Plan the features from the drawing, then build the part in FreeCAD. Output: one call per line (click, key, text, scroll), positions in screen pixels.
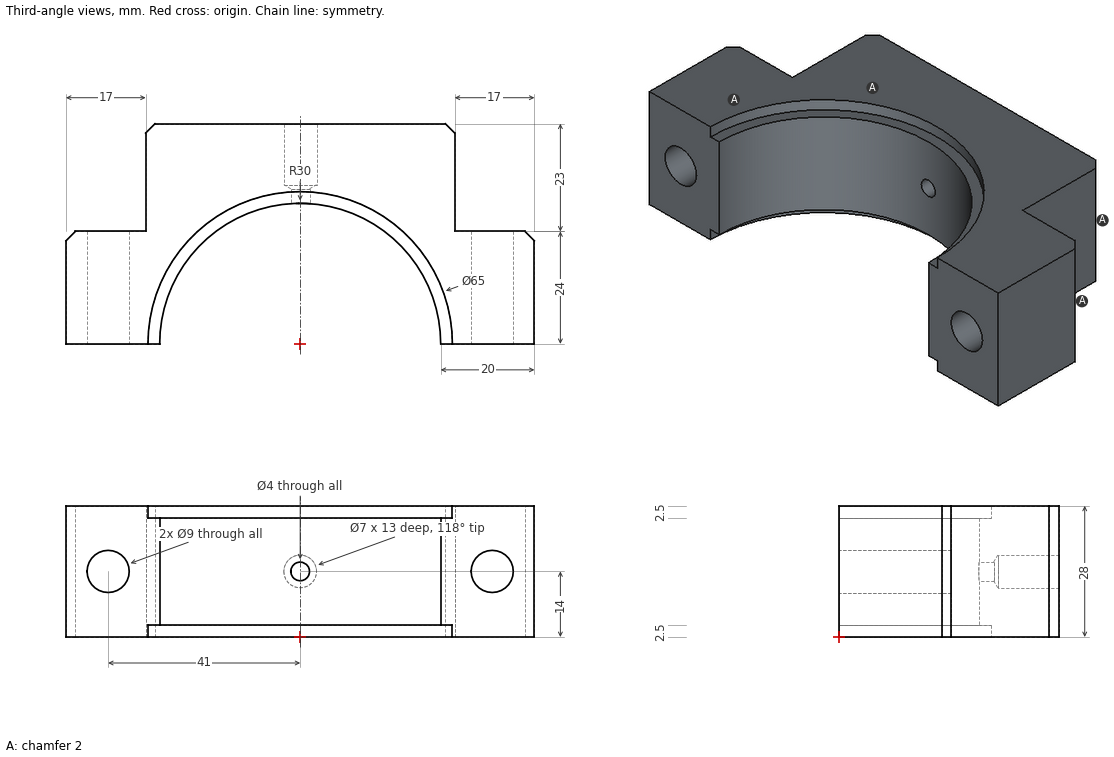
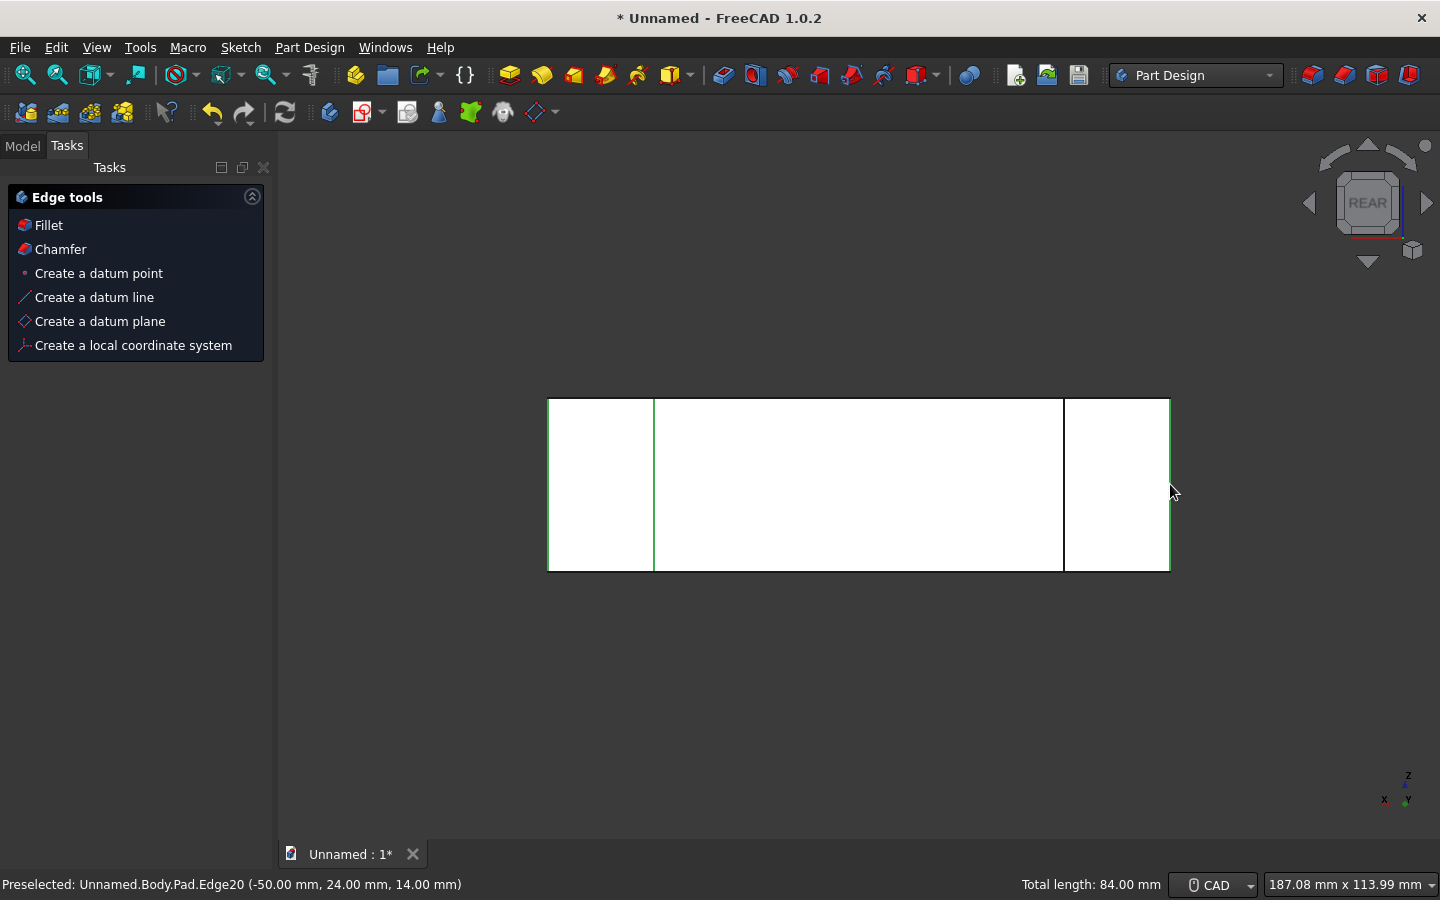
click(1064, 484, ctrl)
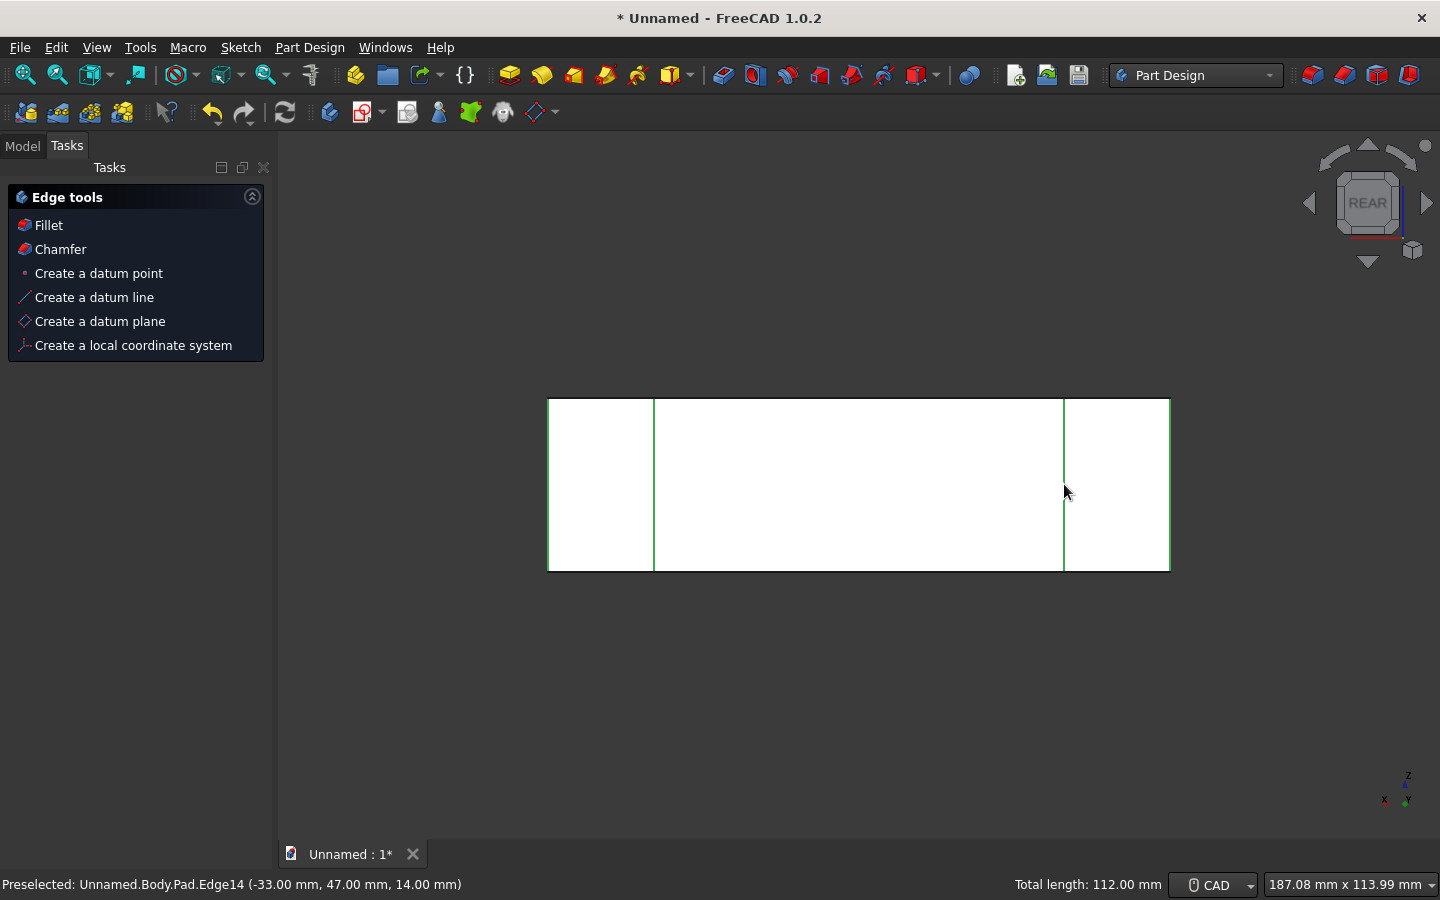
click(1346, 76)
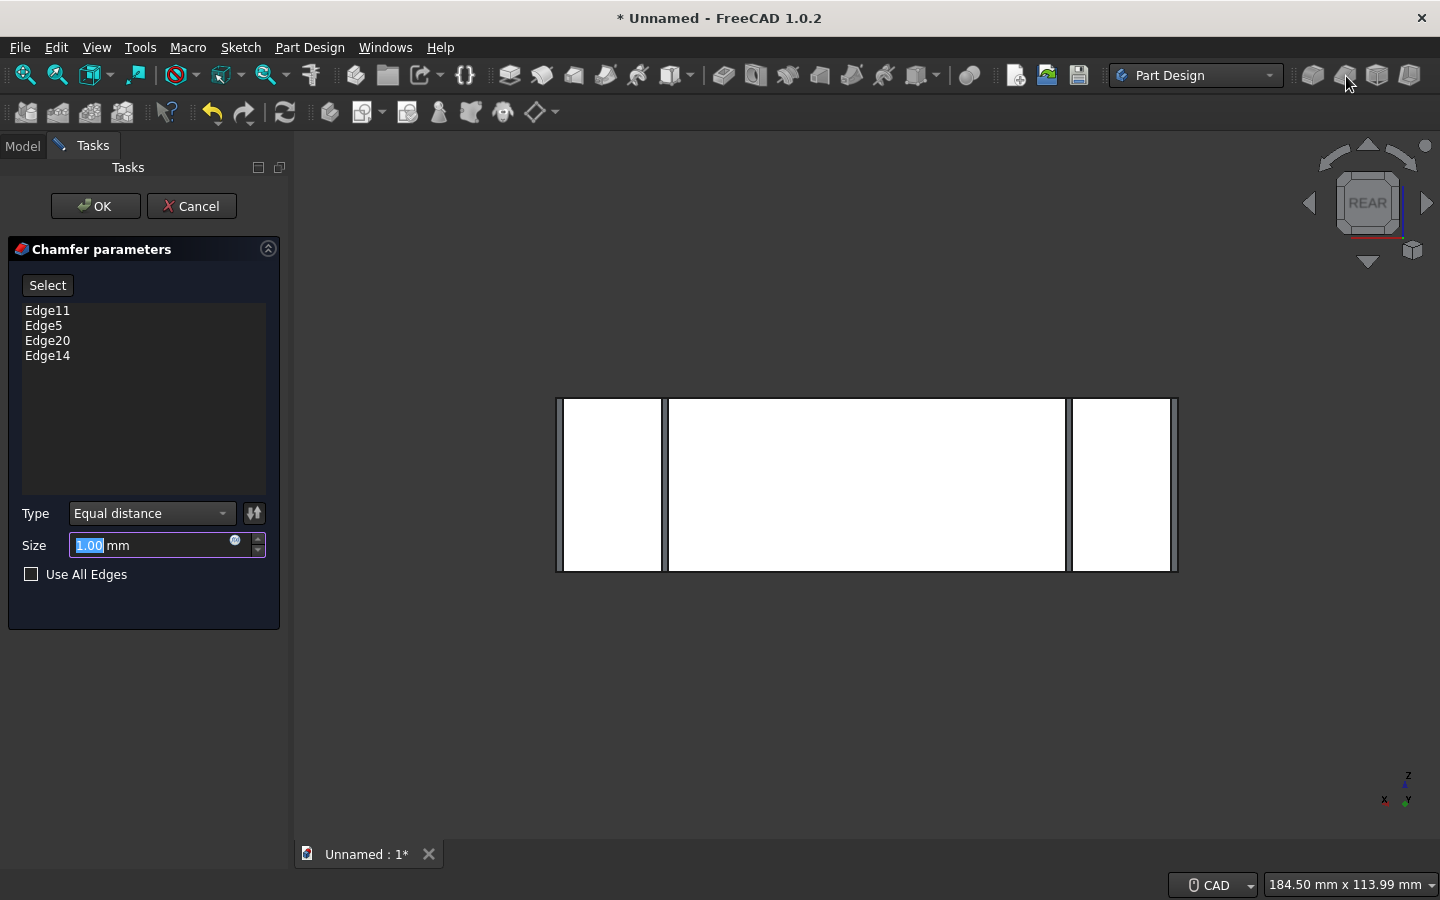
text(2)
key(Tab)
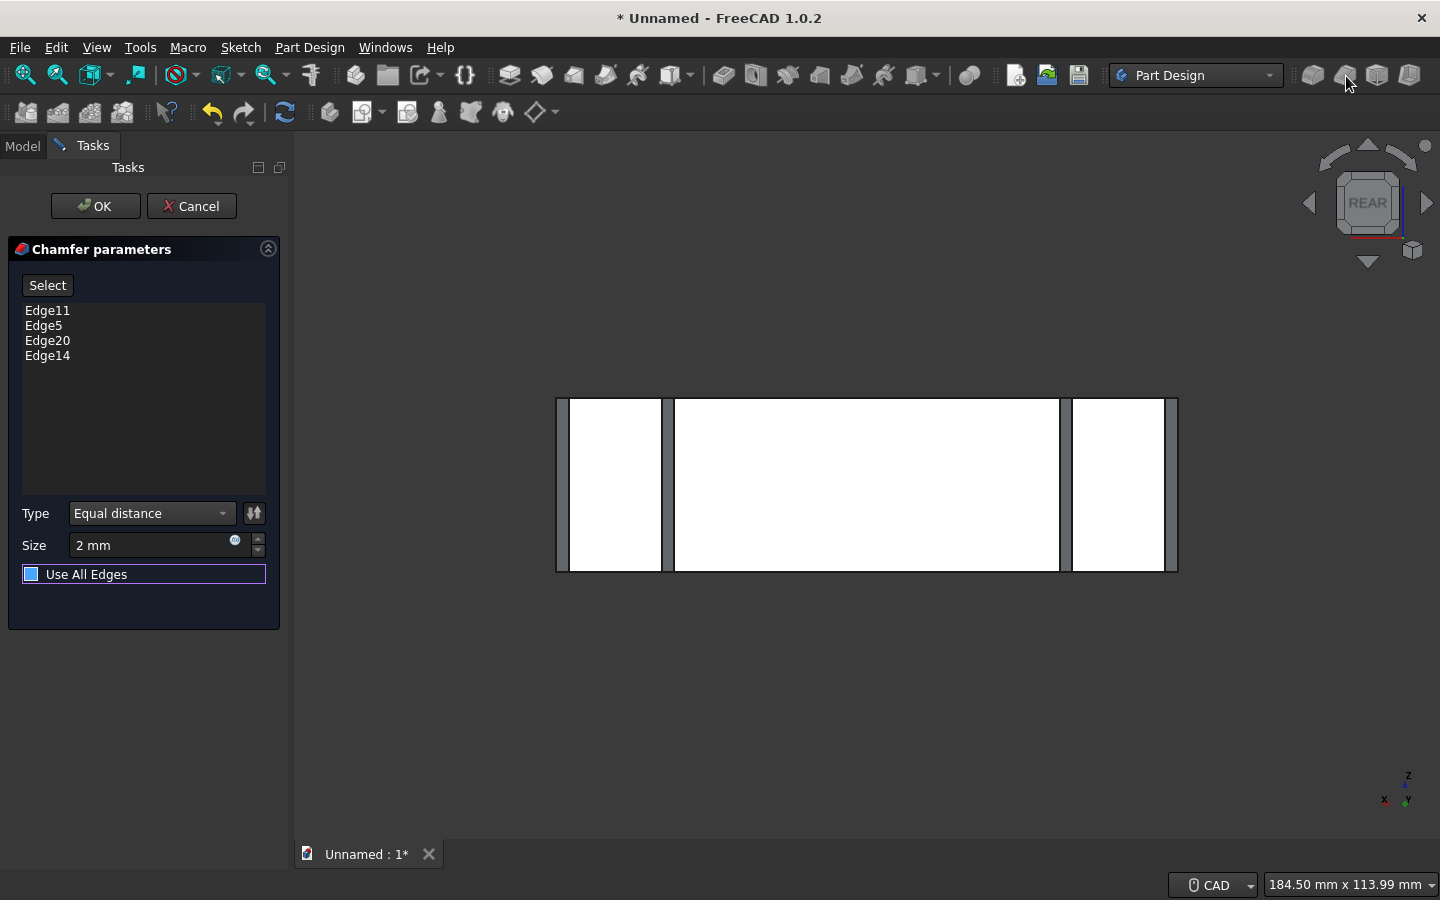
click(96, 206)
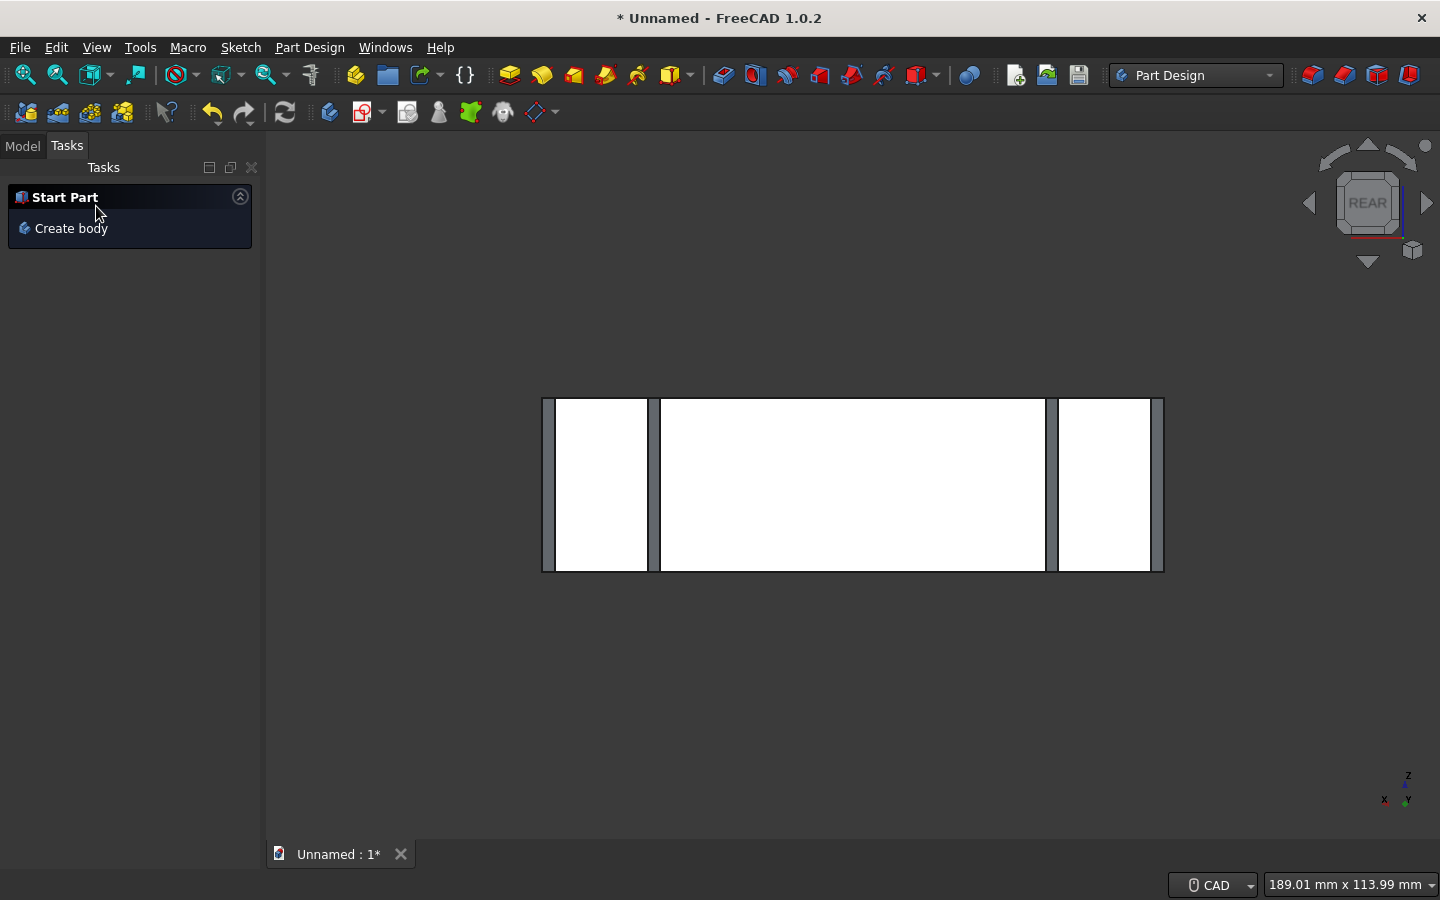
click(798, 484)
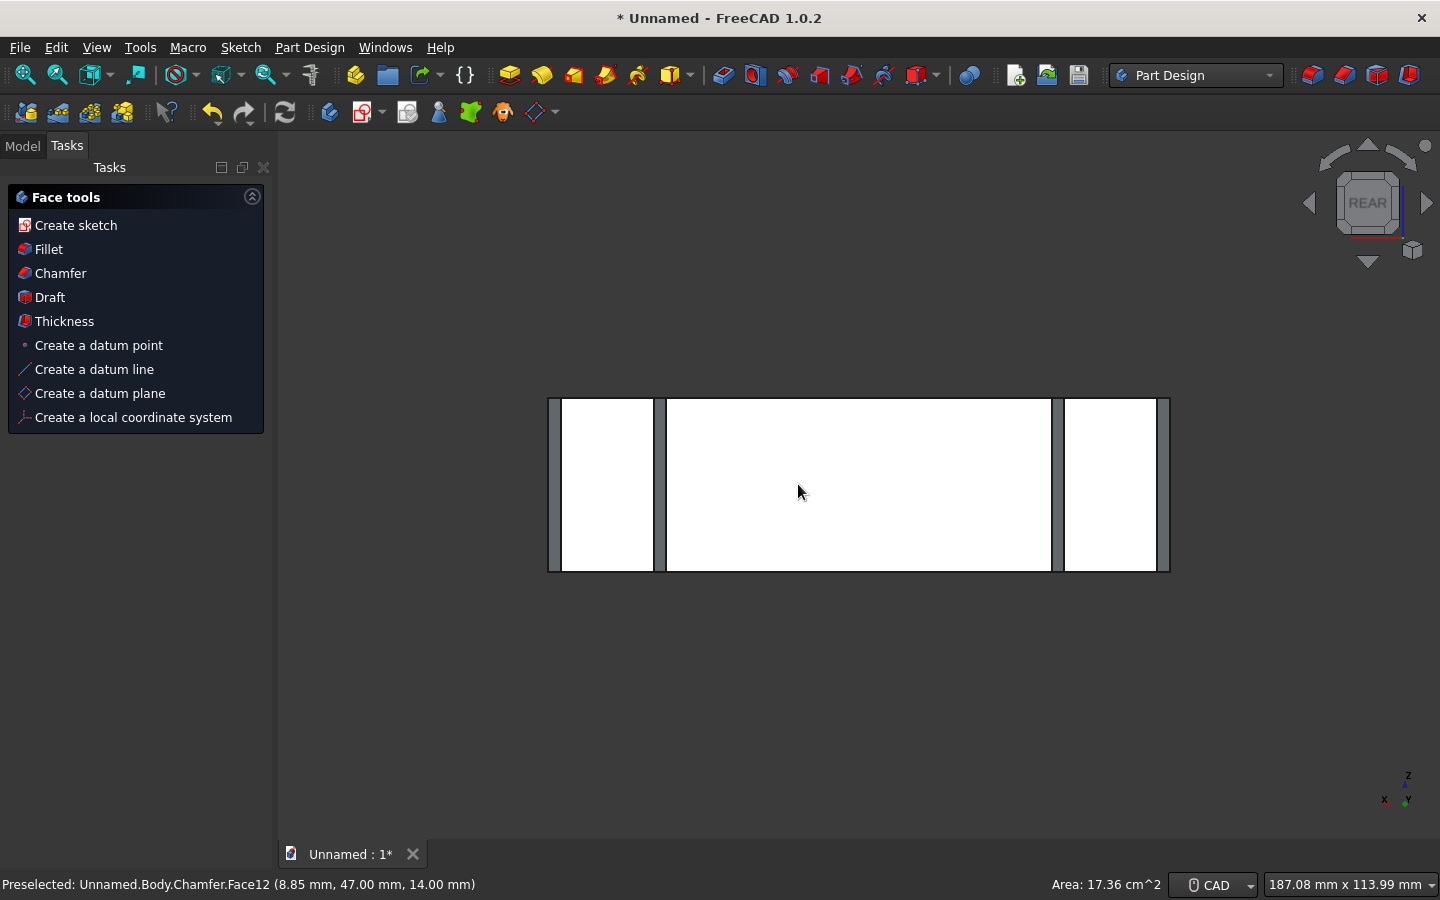
click(362, 112)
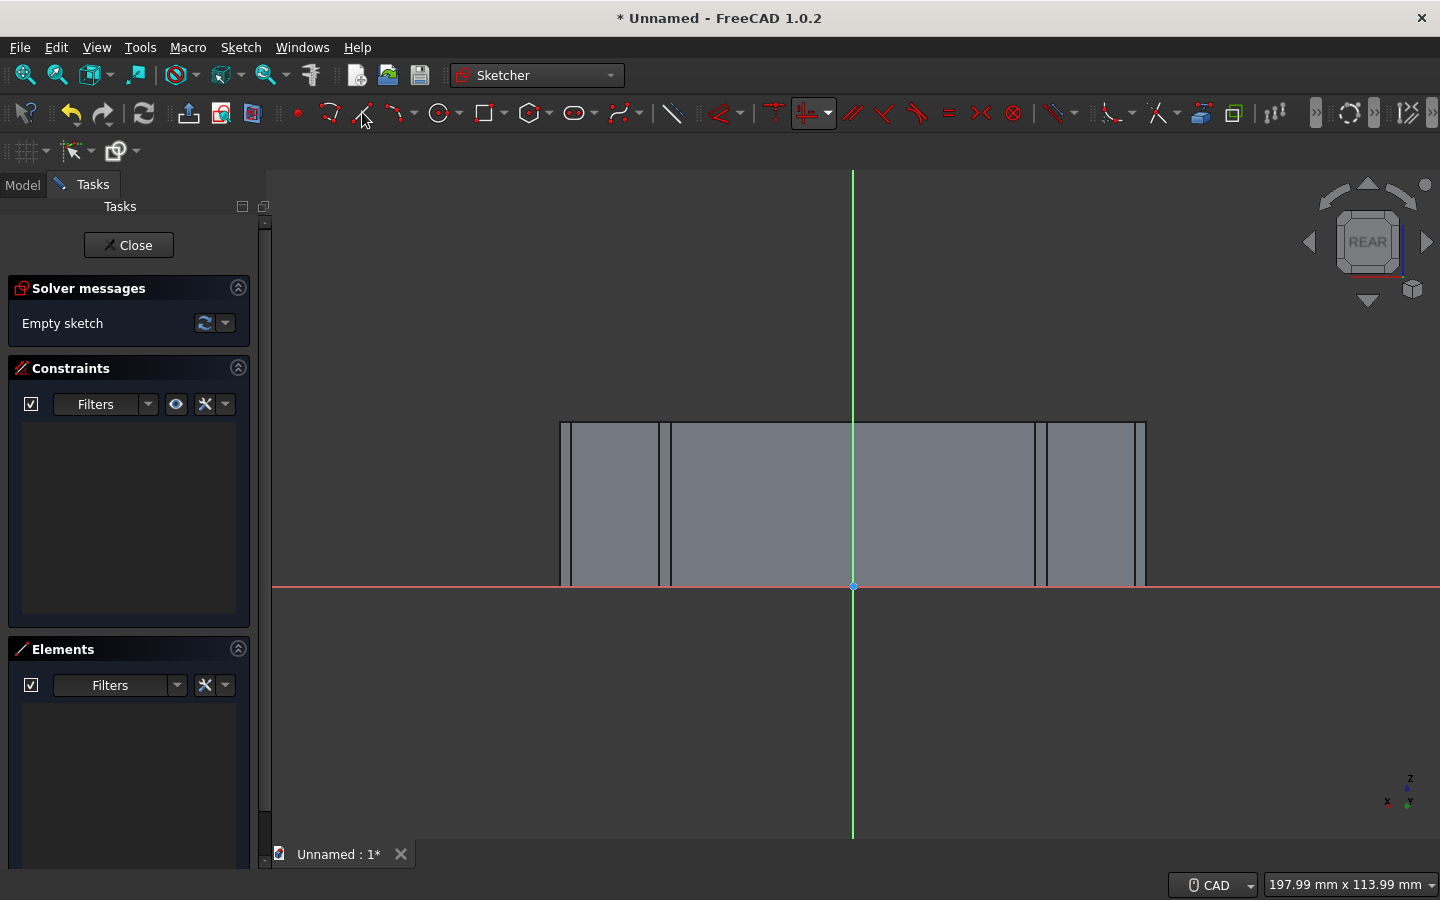
scroll(860, 504, up, 12)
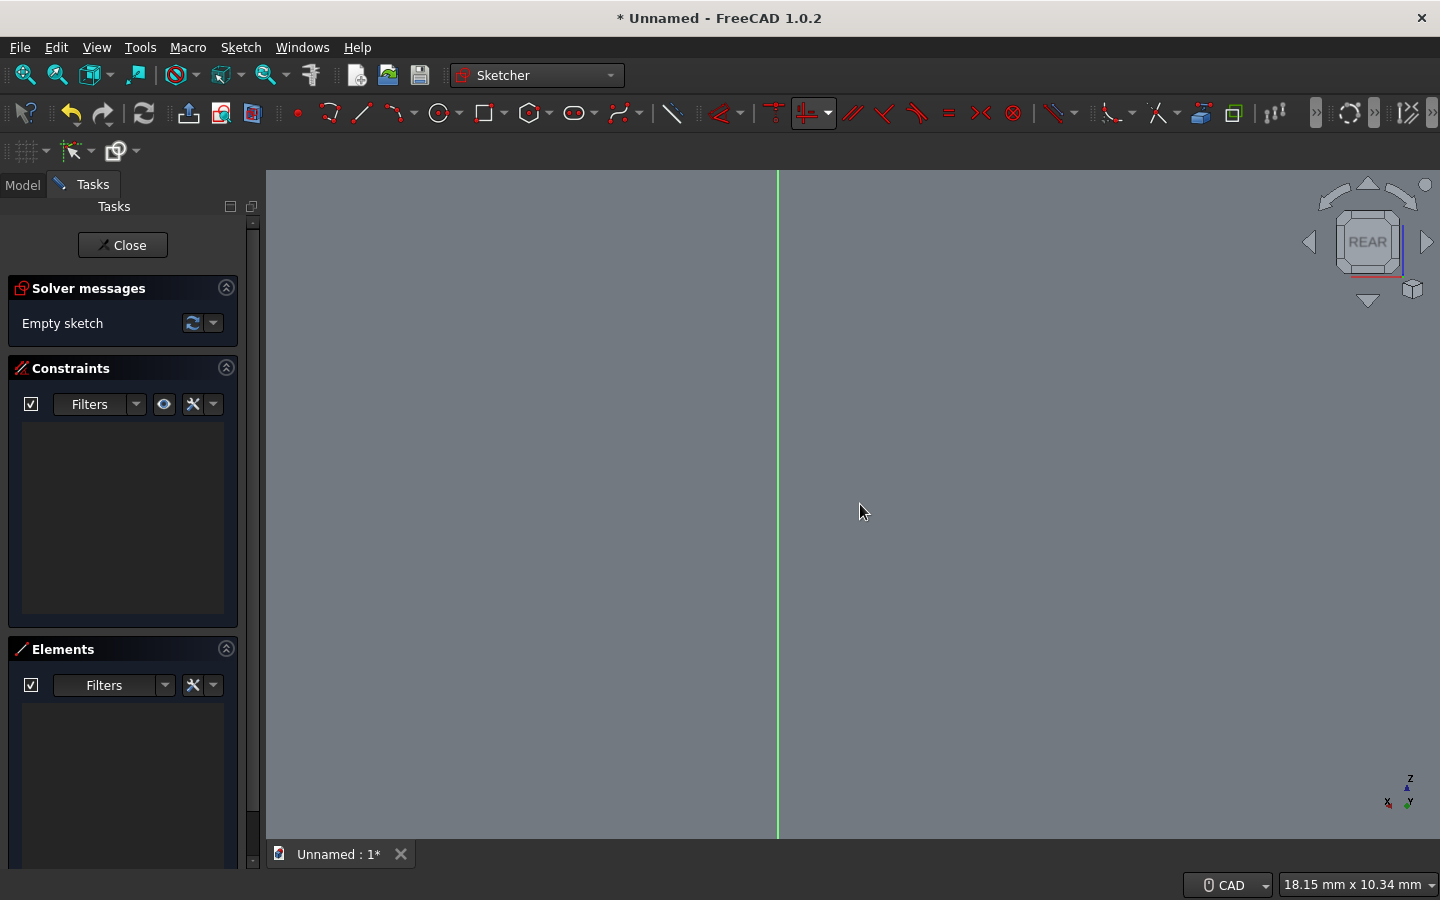
click(440, 114)